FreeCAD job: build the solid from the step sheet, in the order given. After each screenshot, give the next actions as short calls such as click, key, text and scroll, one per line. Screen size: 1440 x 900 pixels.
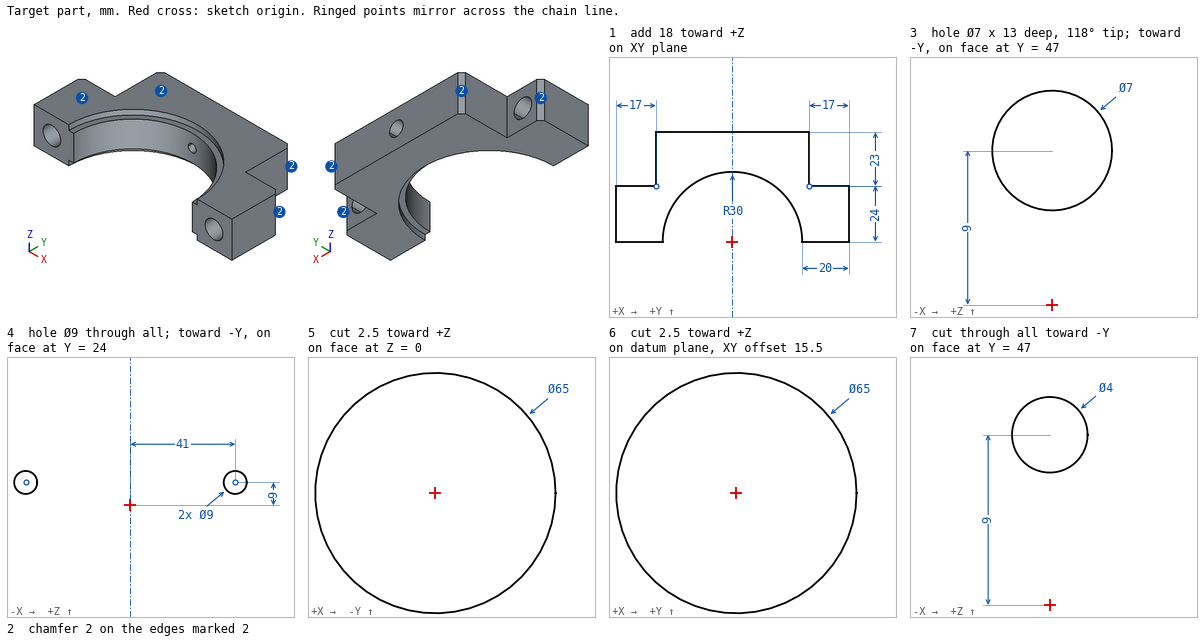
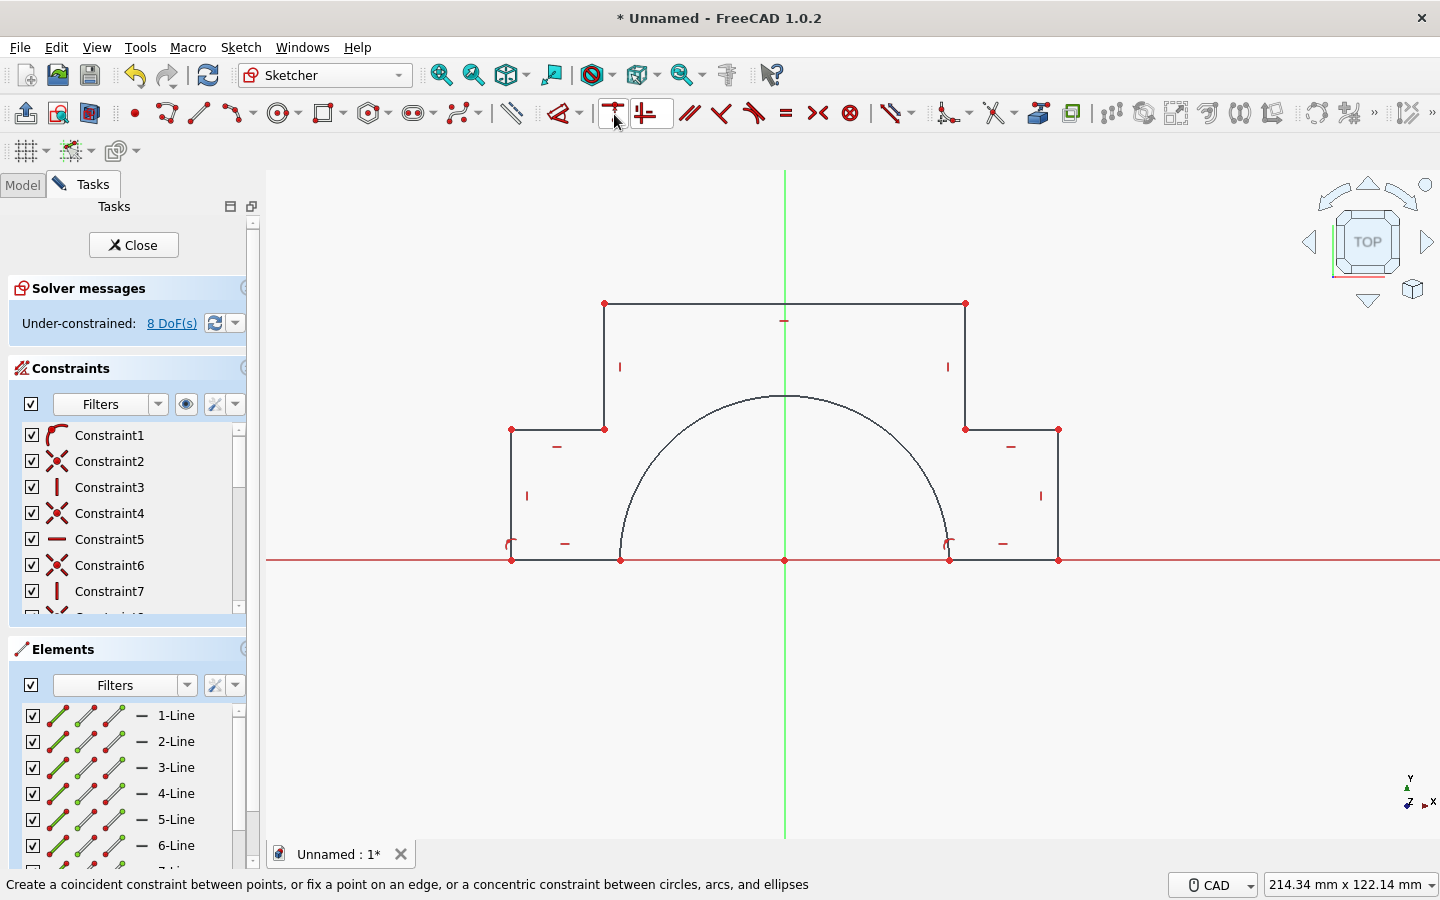
click(965, 430)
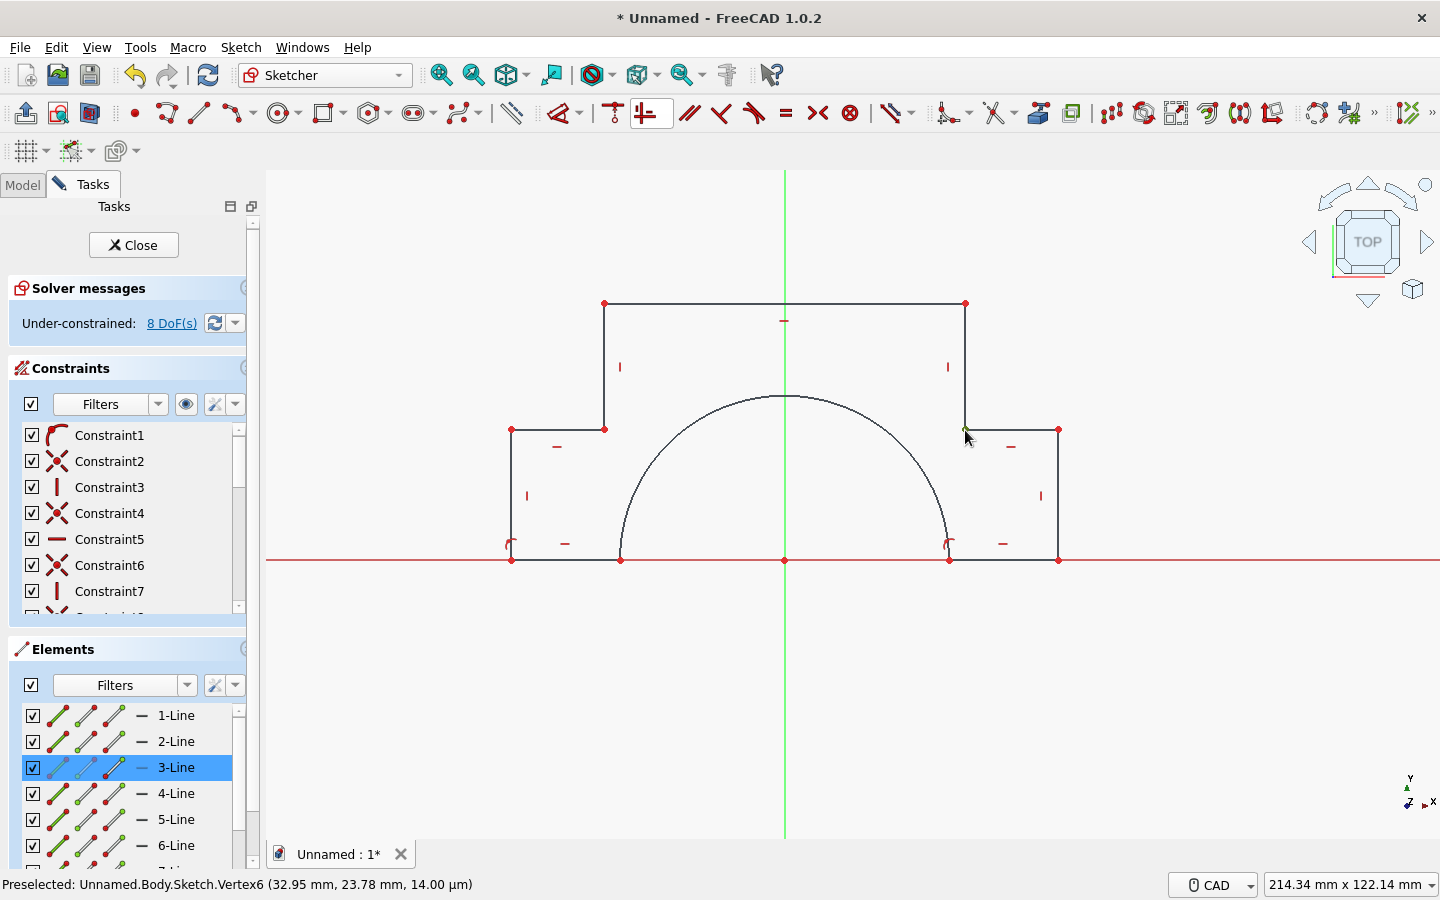
click(604, 430)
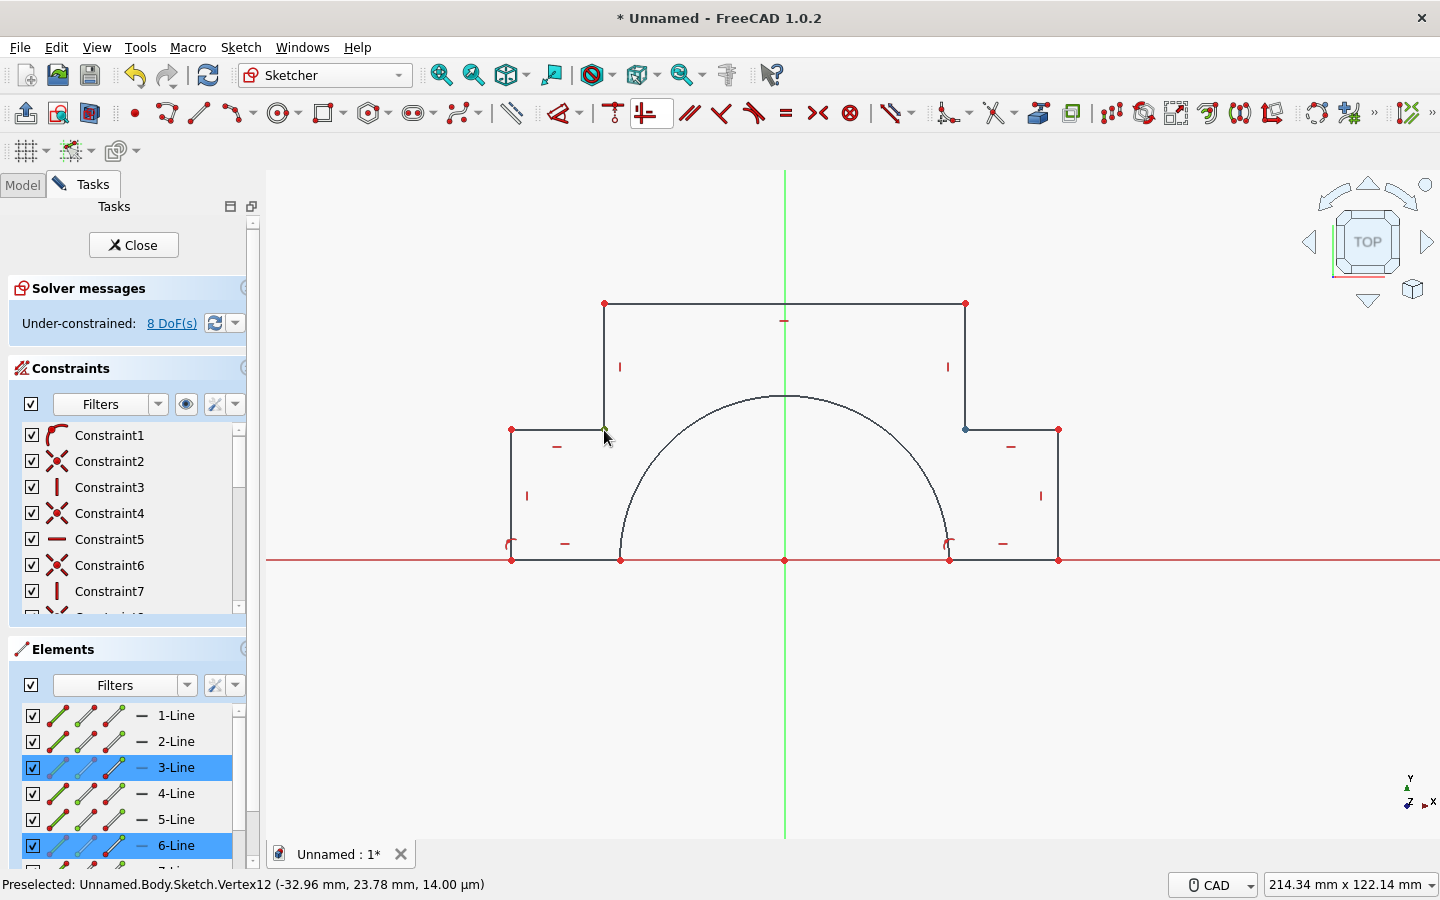
click(785, 767)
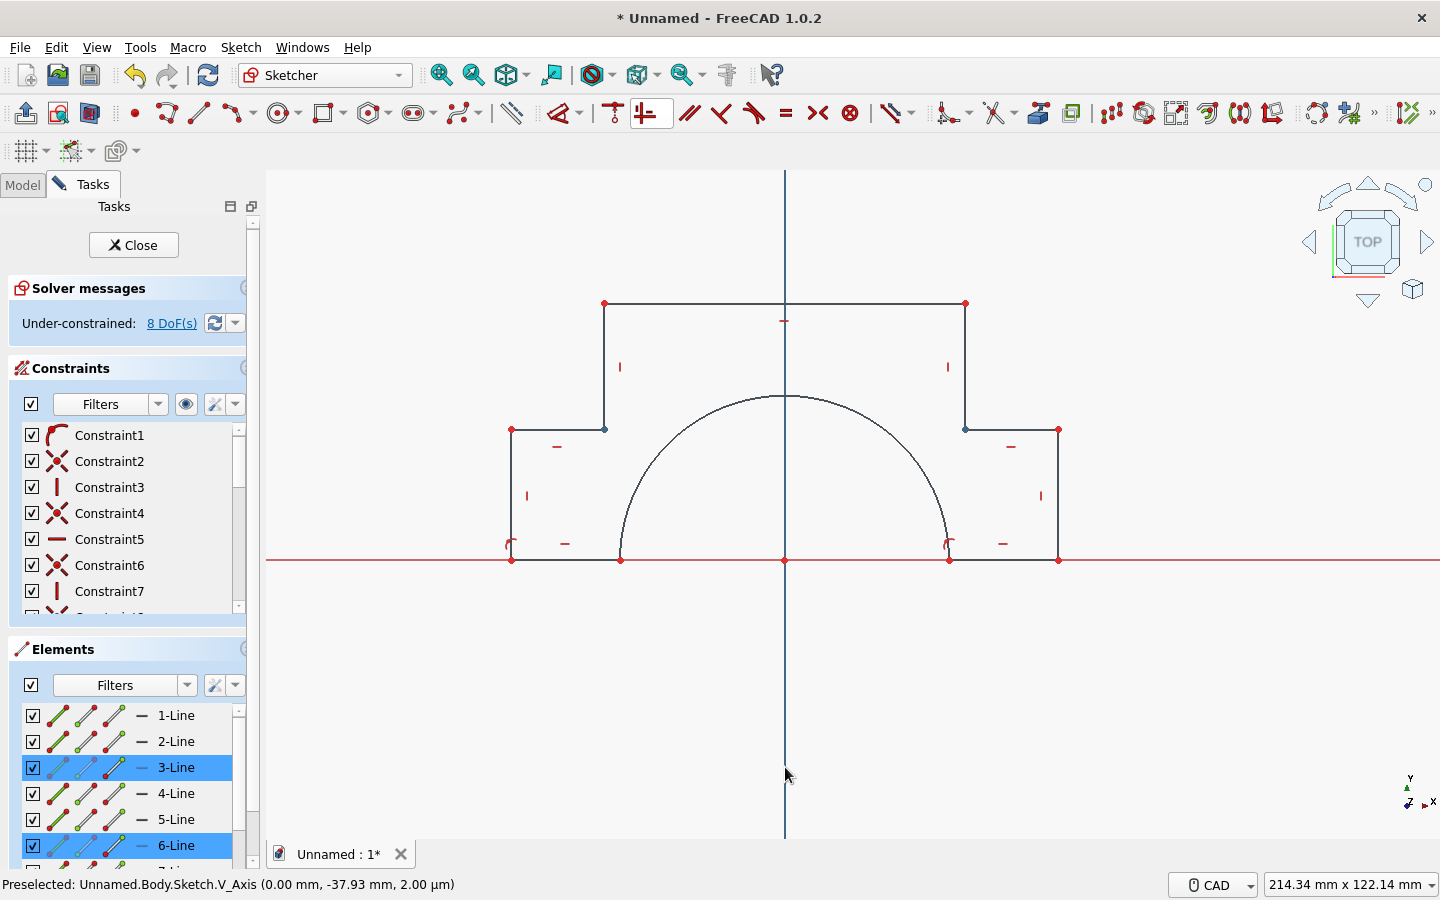
click(818, 114)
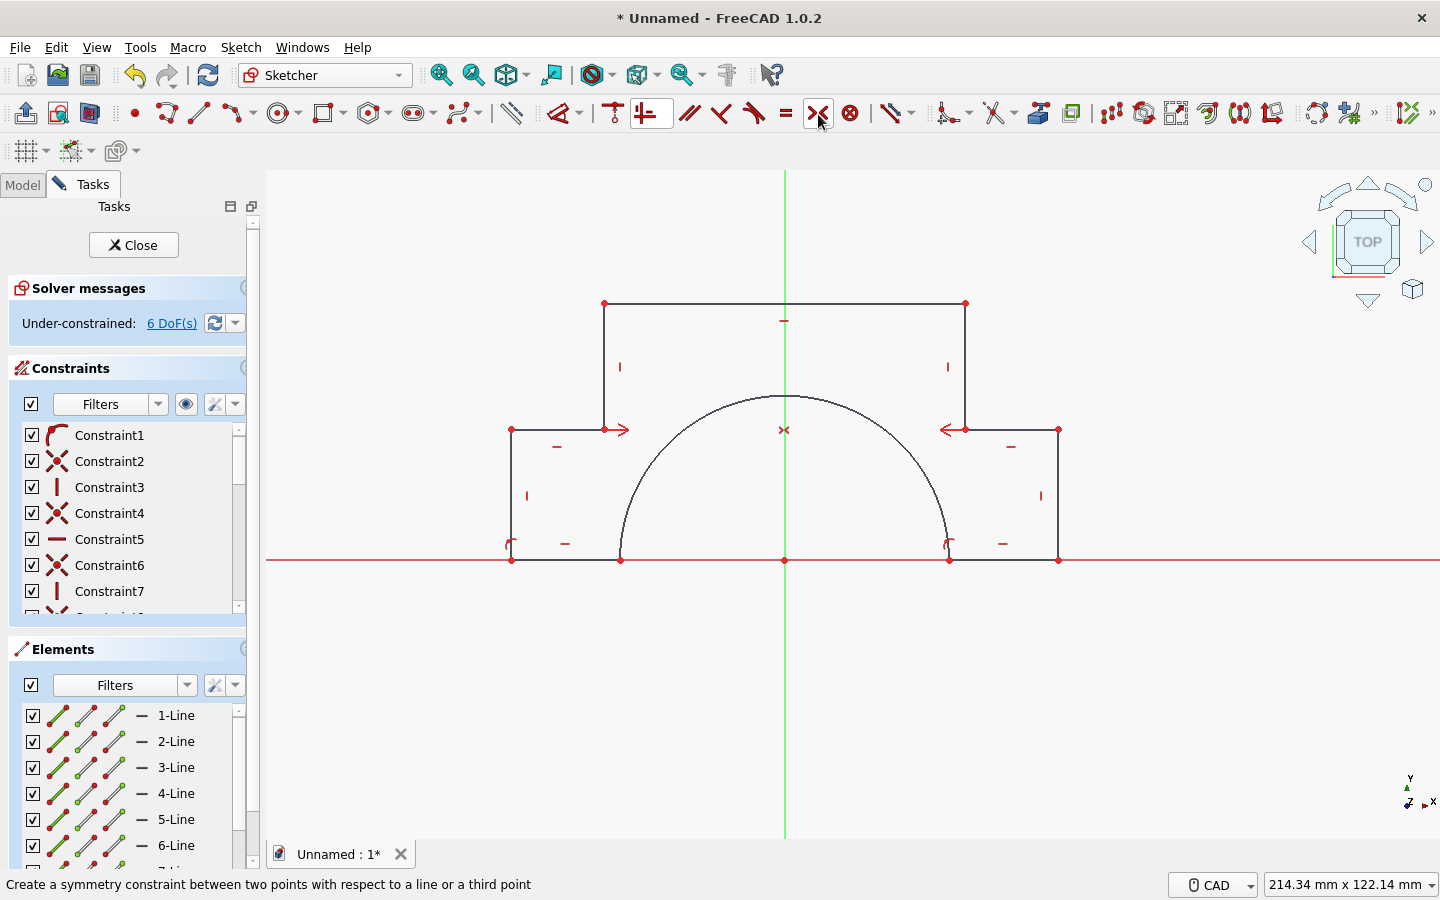
click(881, 427)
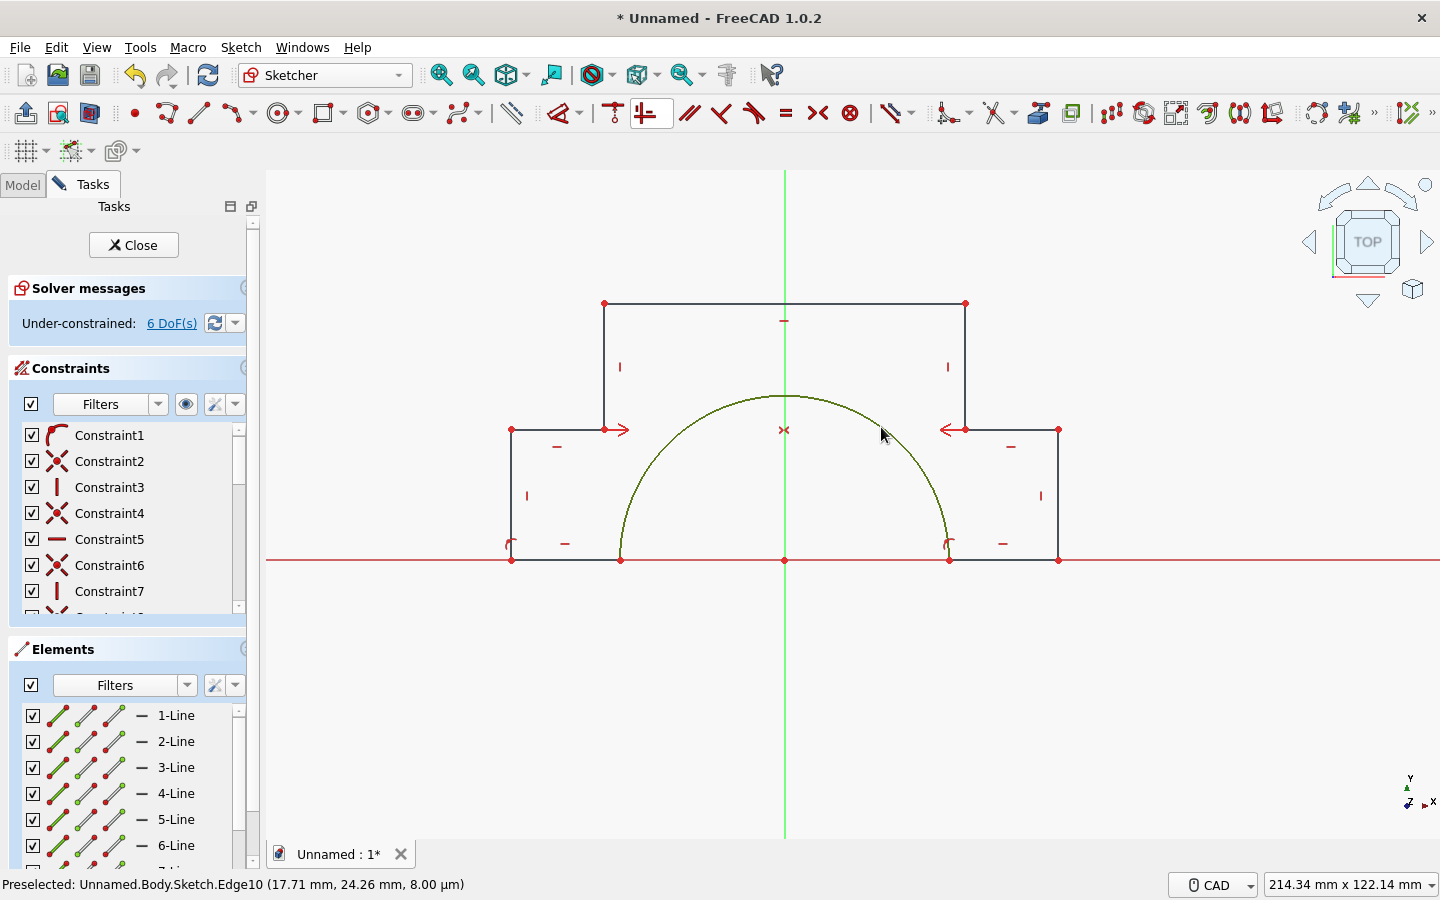
click(582, 114)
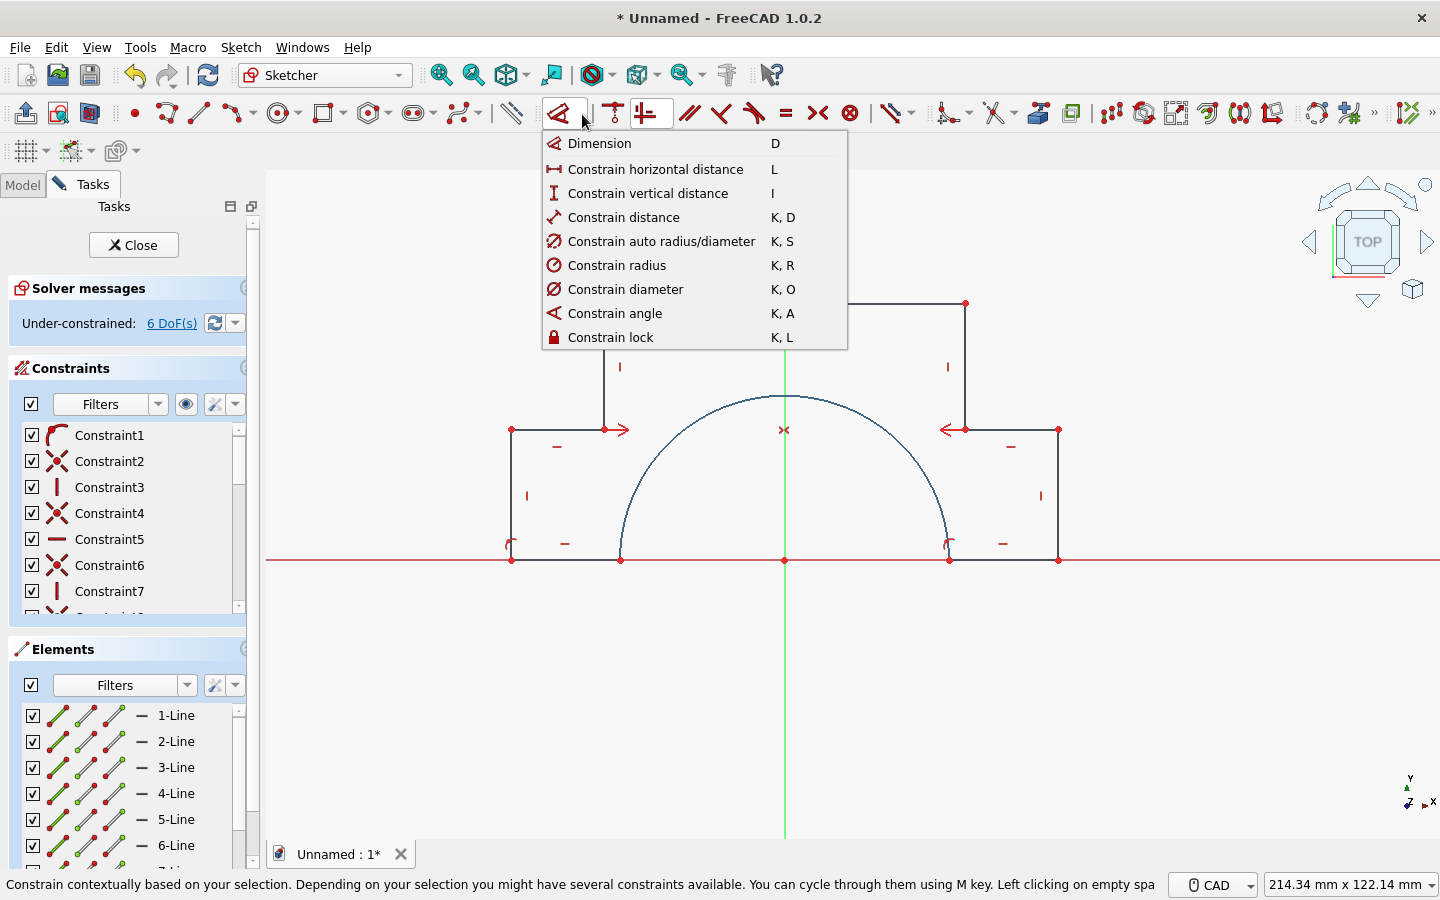
click(695, 265)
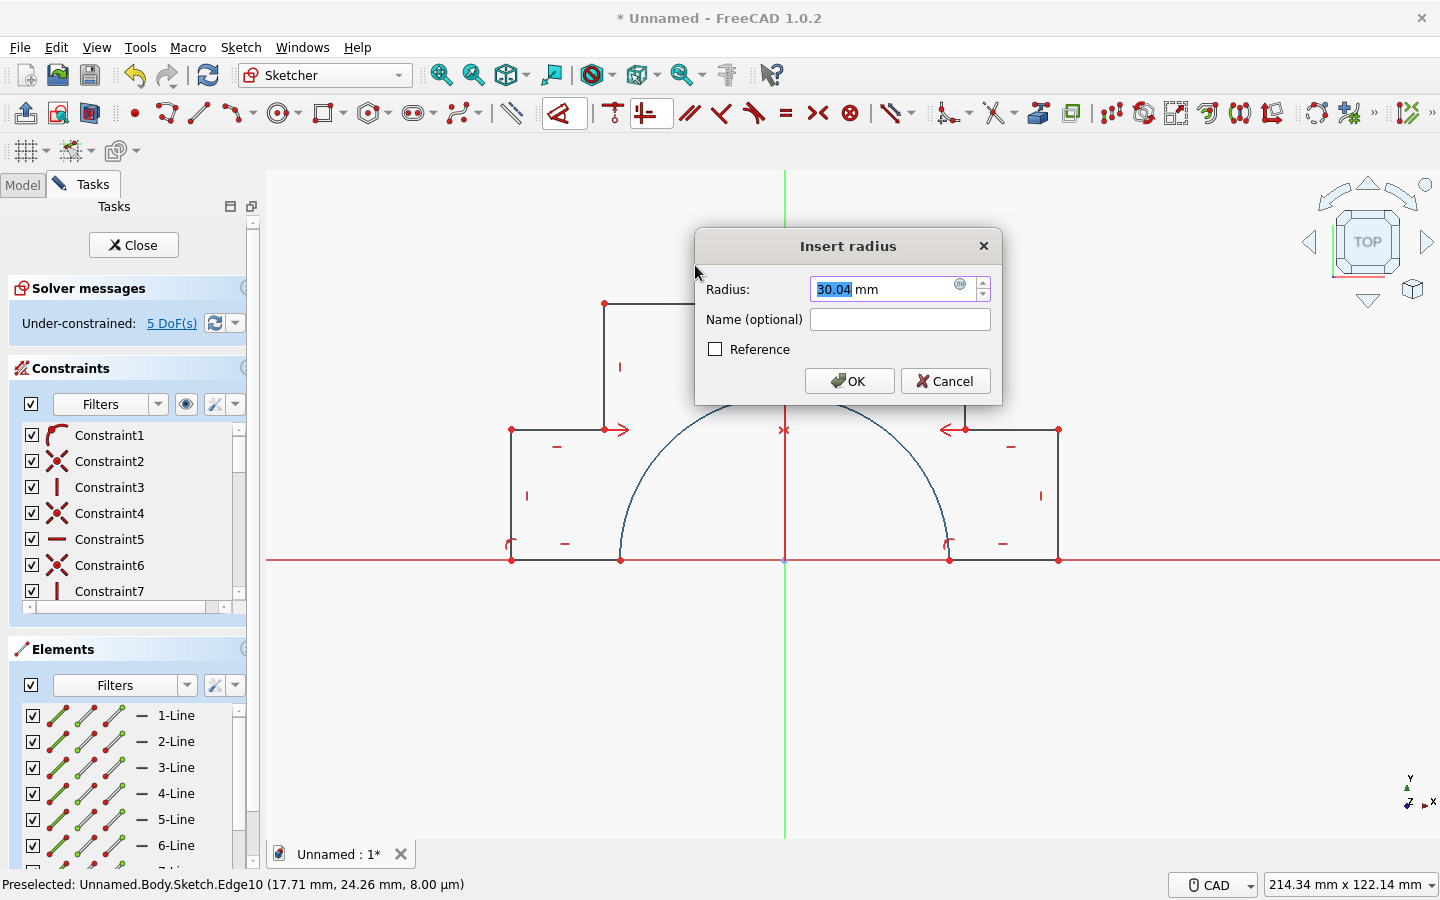
text(30)
key(Return)